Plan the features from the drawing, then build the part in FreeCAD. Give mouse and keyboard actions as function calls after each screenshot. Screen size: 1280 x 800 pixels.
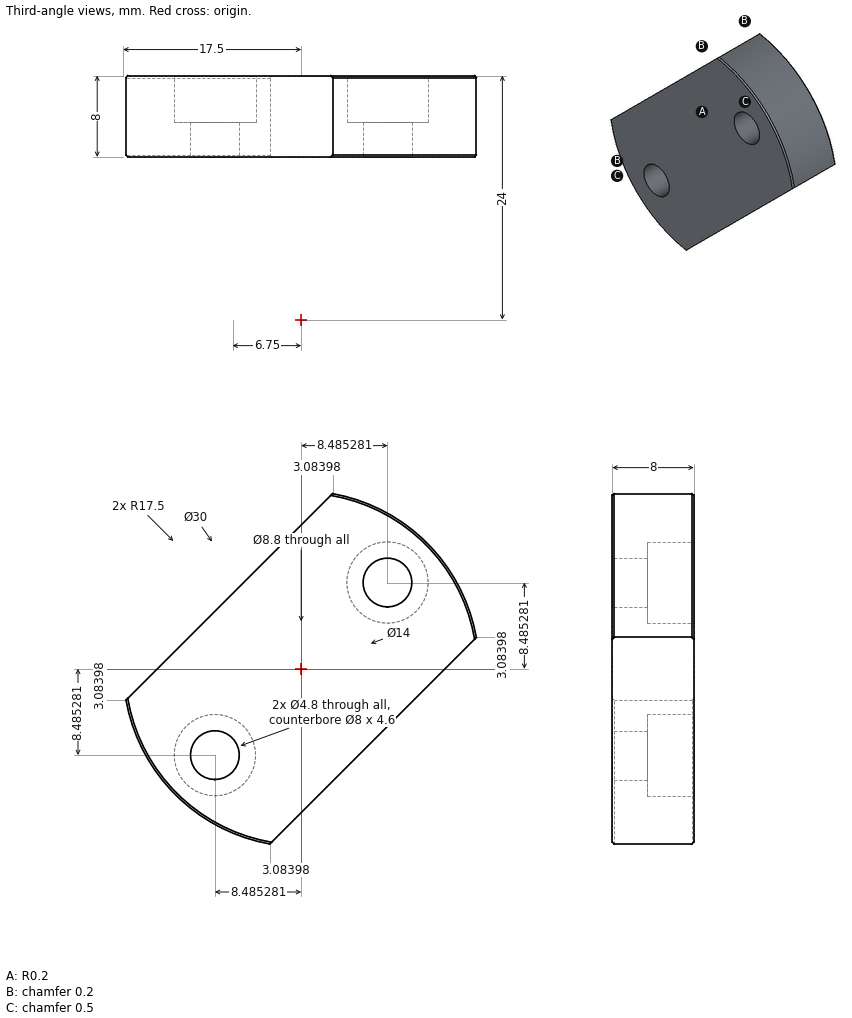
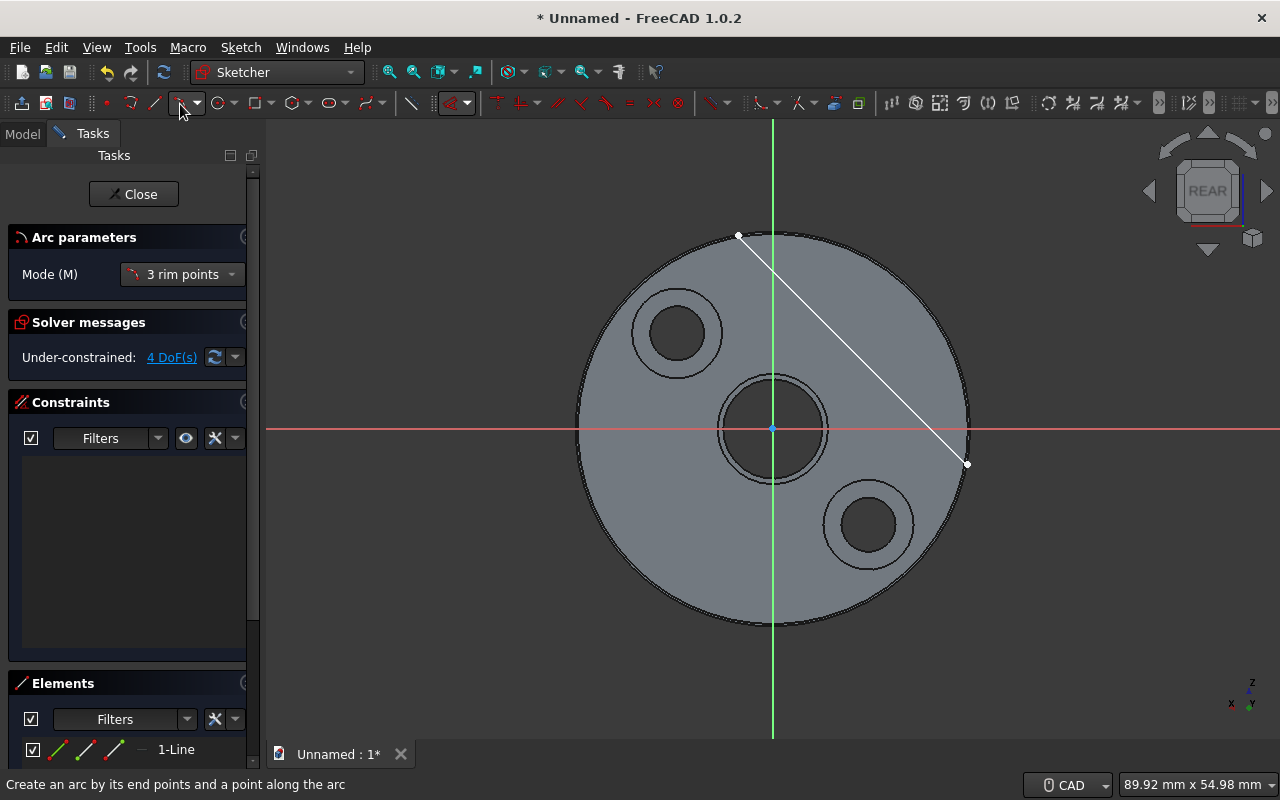
click(967, 465)
click(738, 236)
click(912, 289)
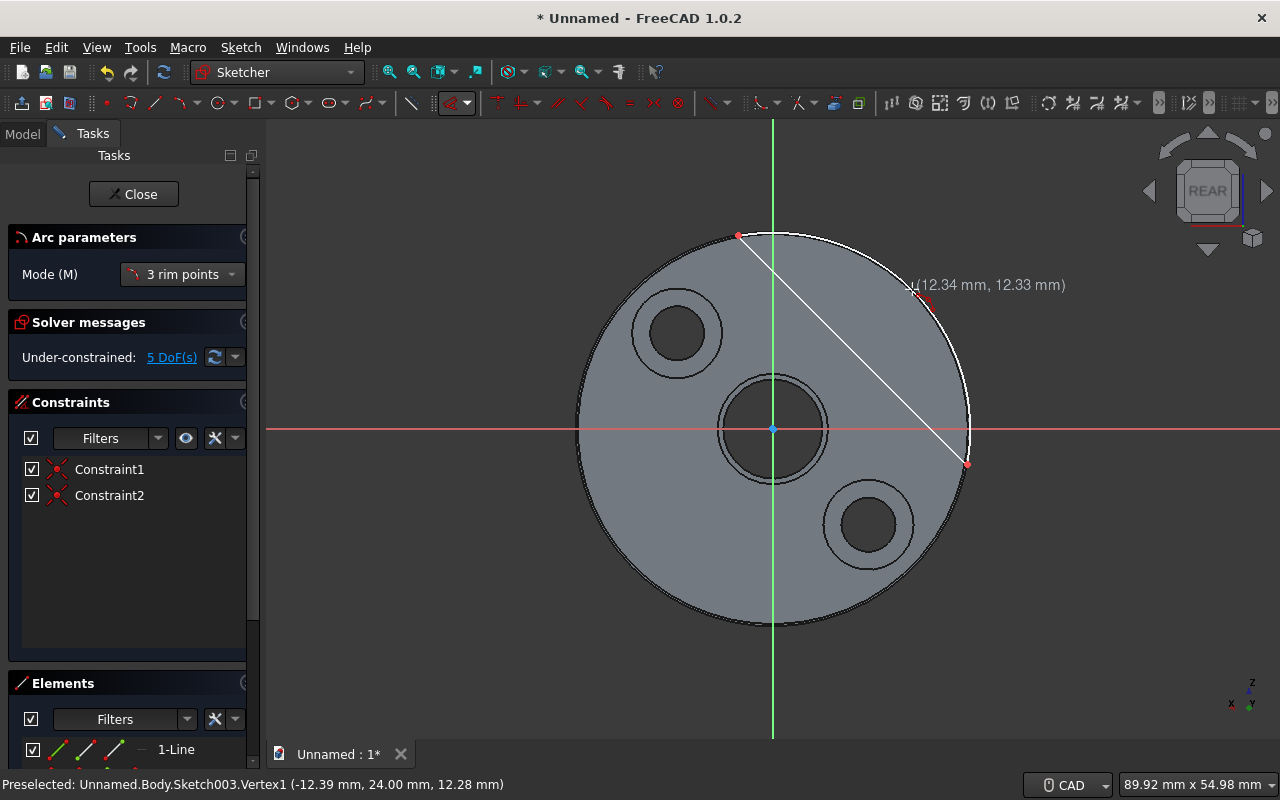
click(156, 104)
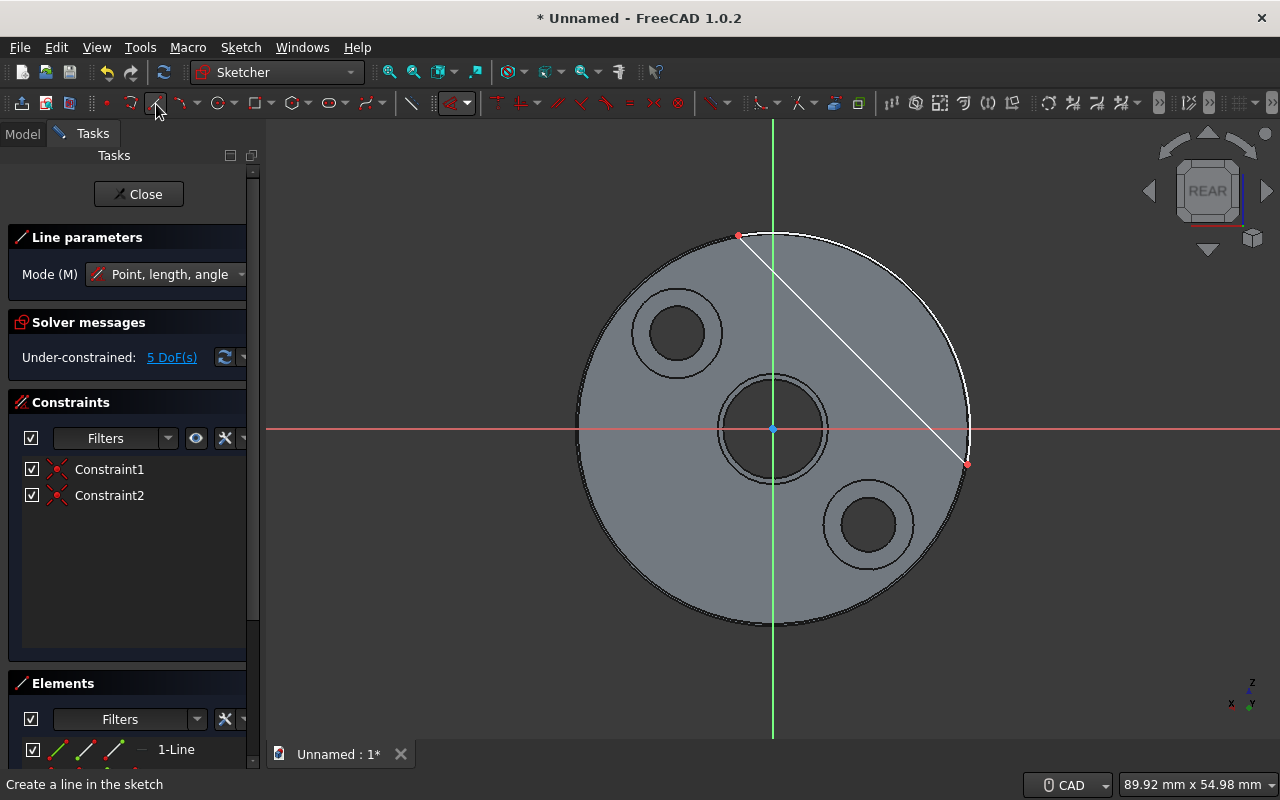
click(808, 623)
click(579, 394)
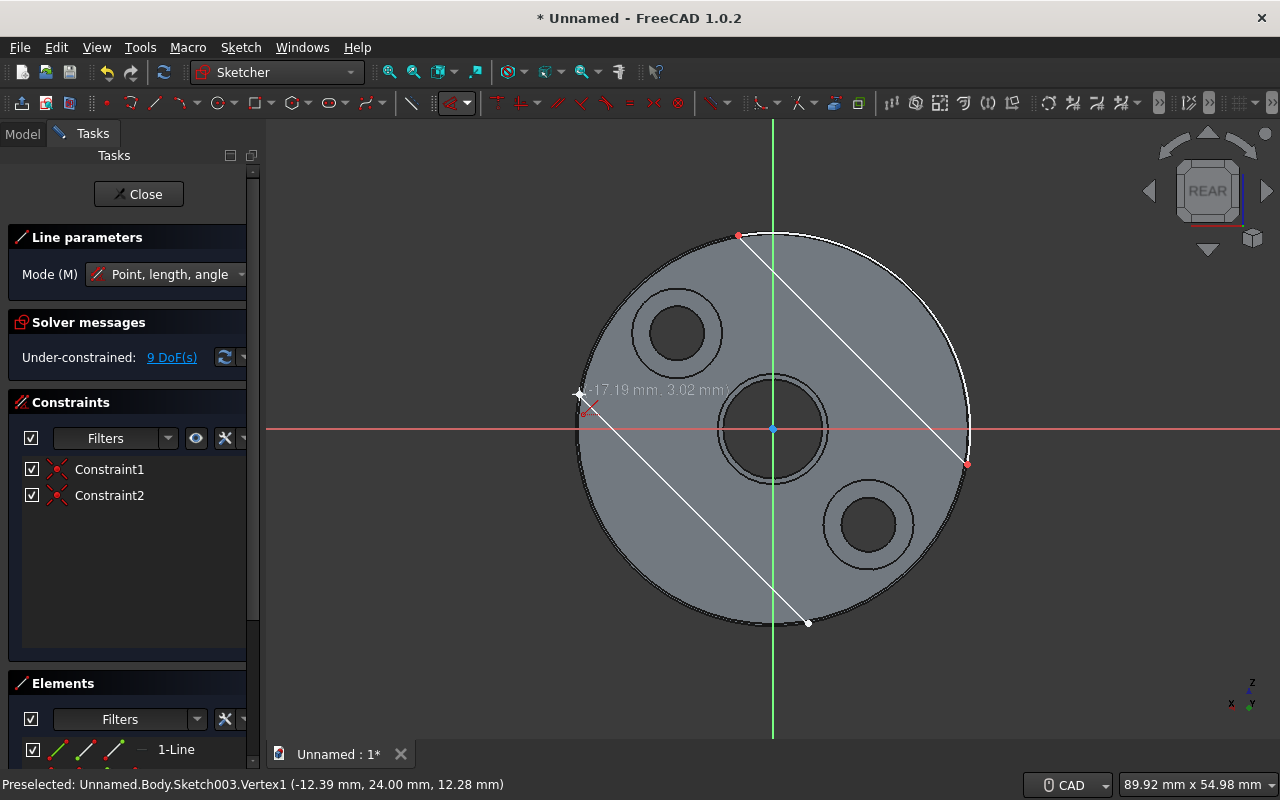
click(180, 104)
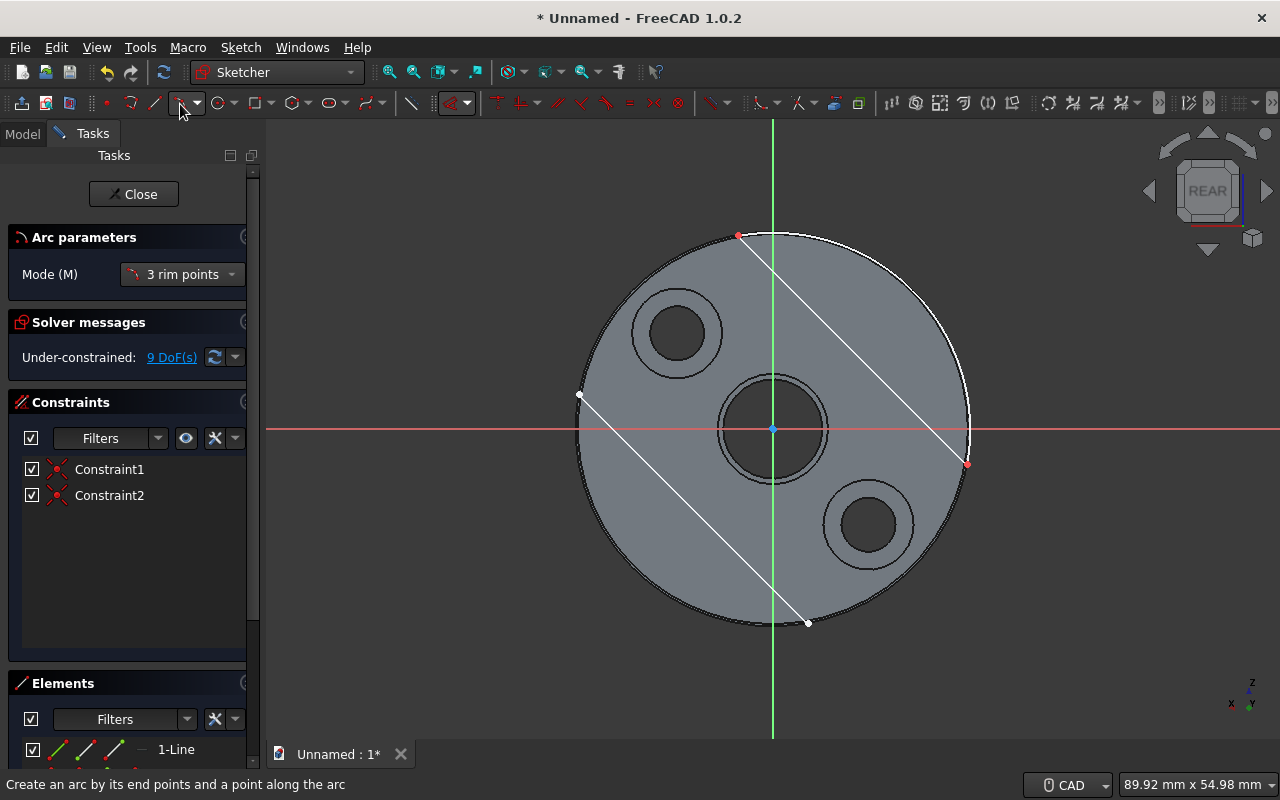
click(579, 395)
click(808, 624)
click(633, 569)
key(Escape)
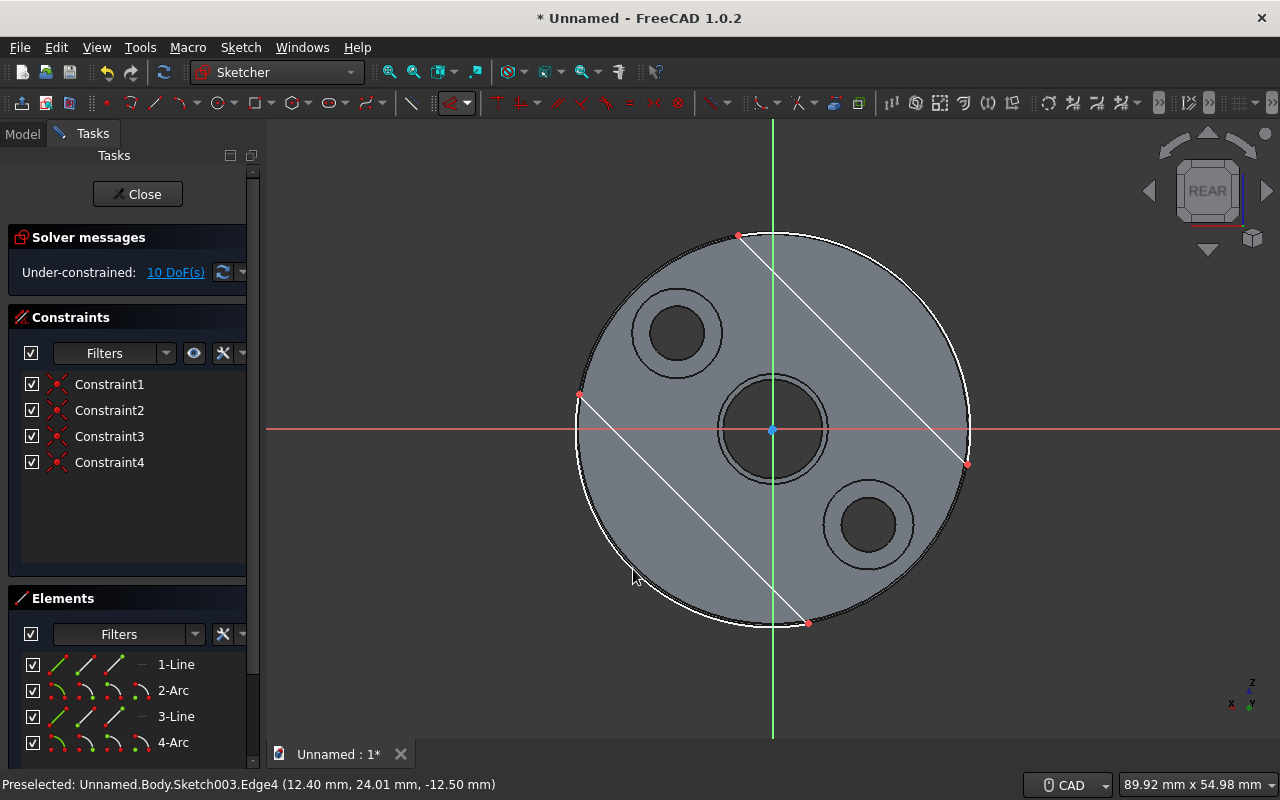
click(955, 353)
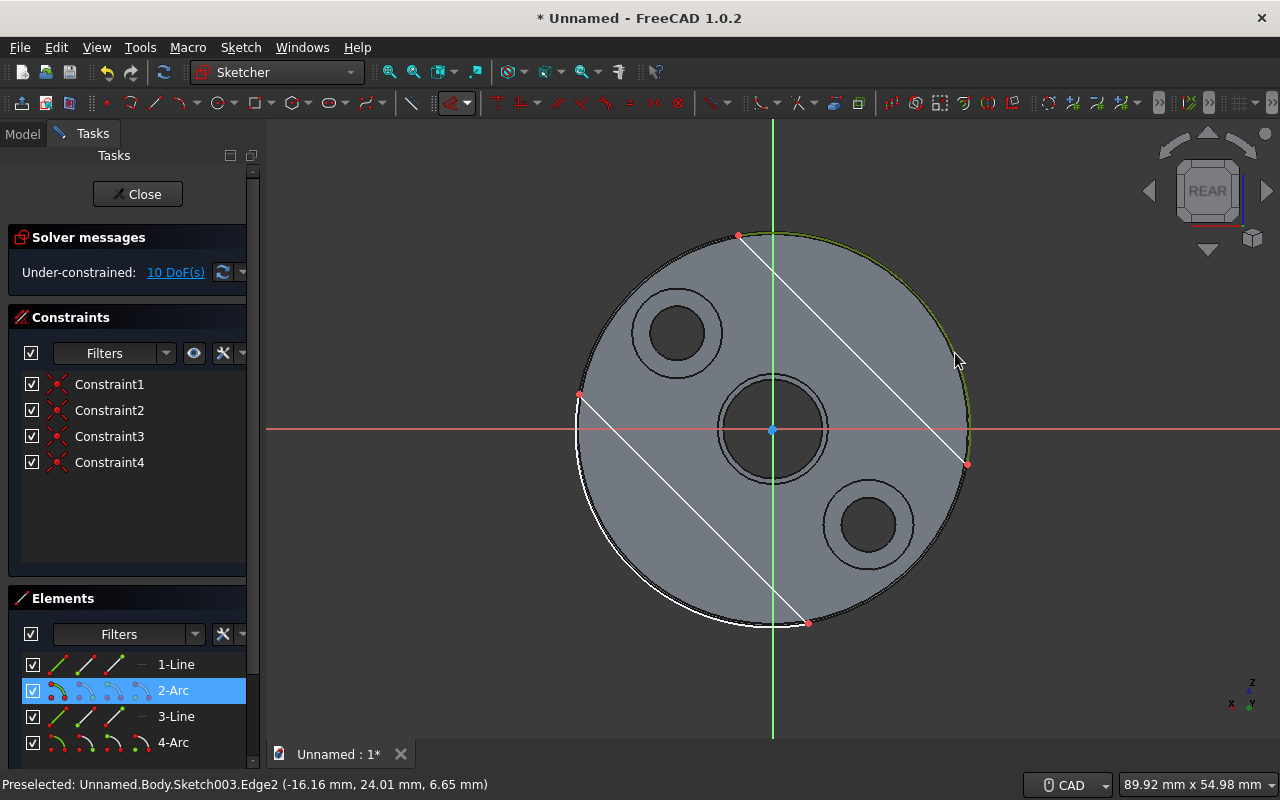
click(591, 507)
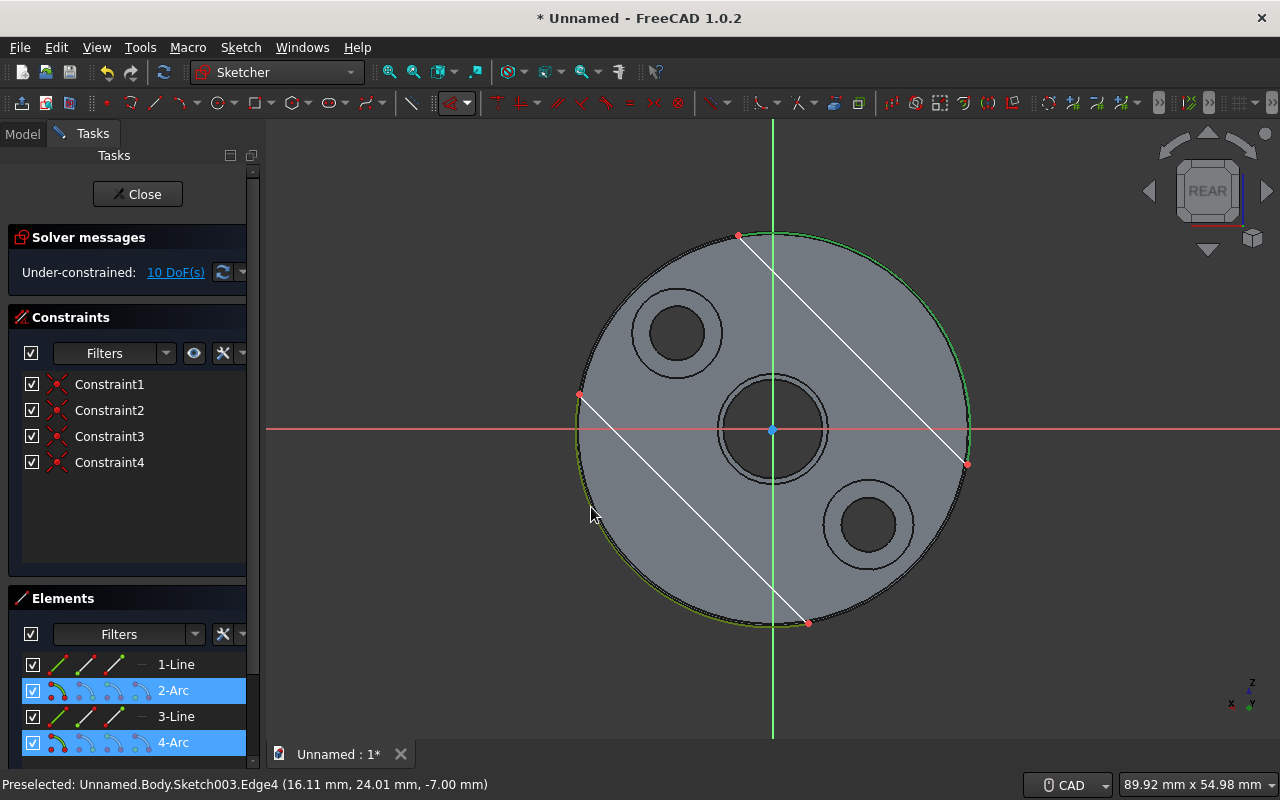
click(498, 104)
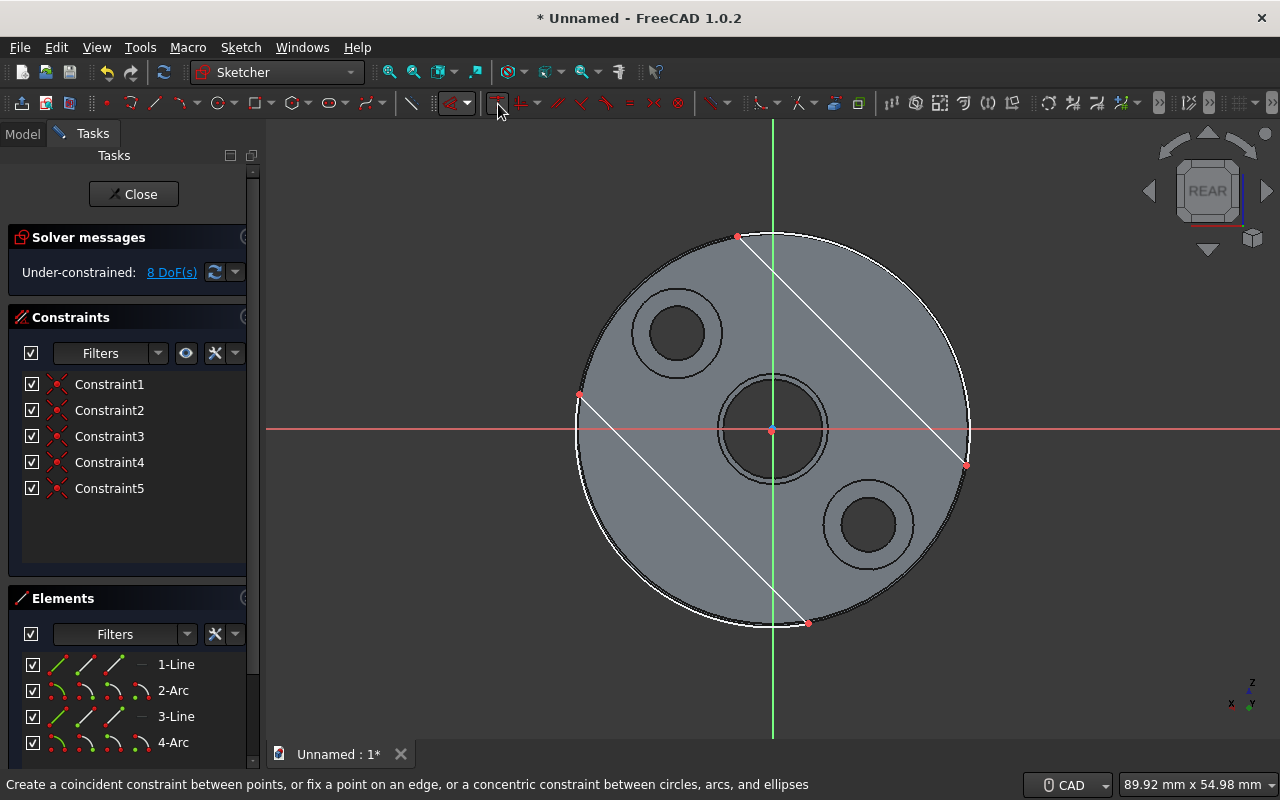
drag(762, 419, 783, 441)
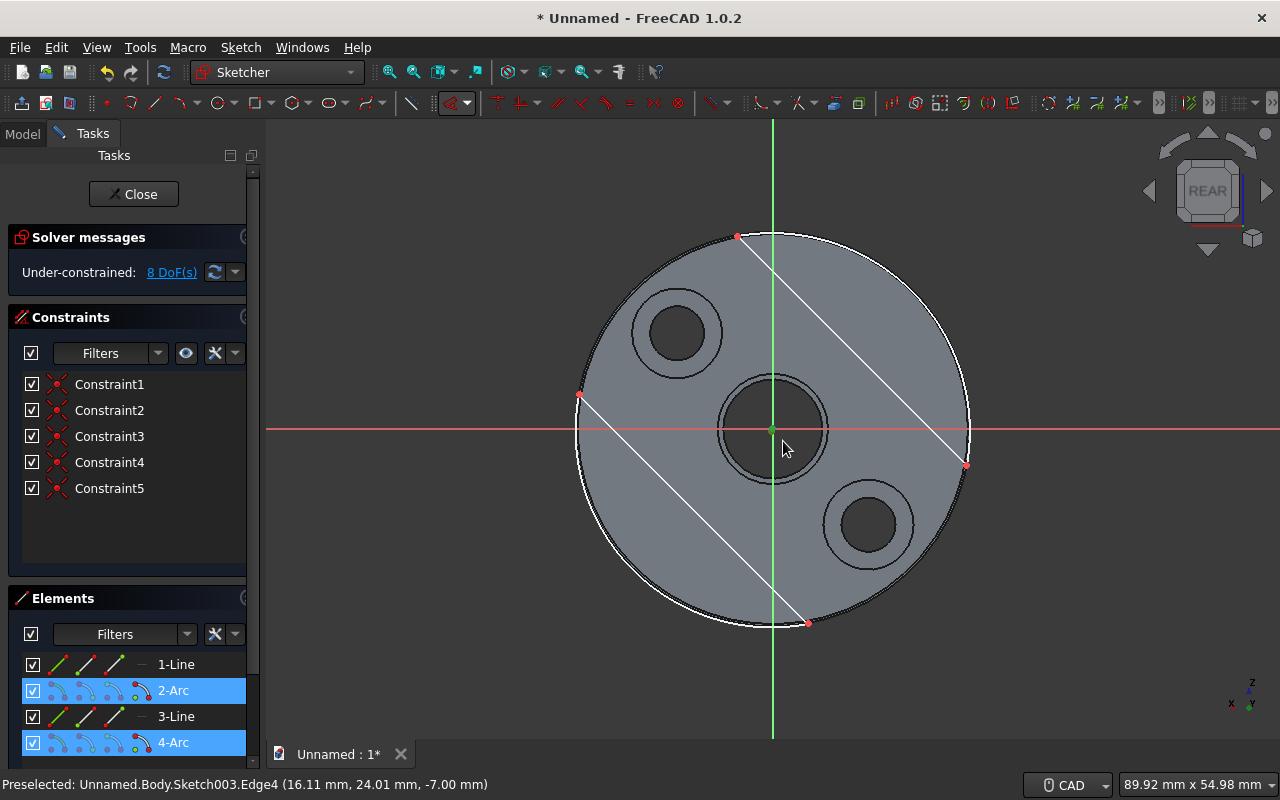
click(498, 104)